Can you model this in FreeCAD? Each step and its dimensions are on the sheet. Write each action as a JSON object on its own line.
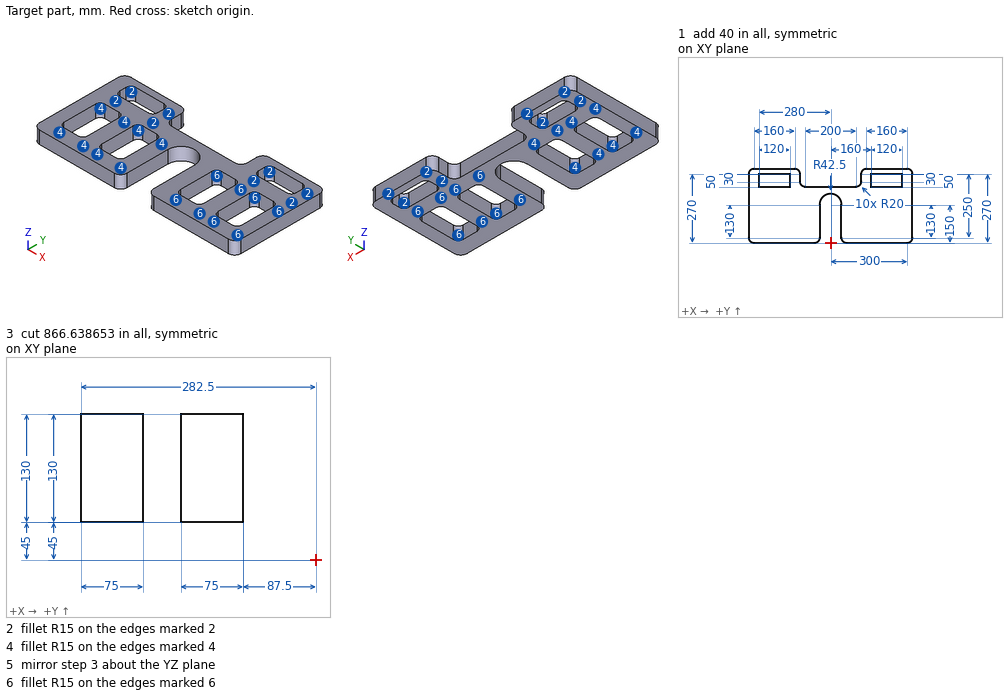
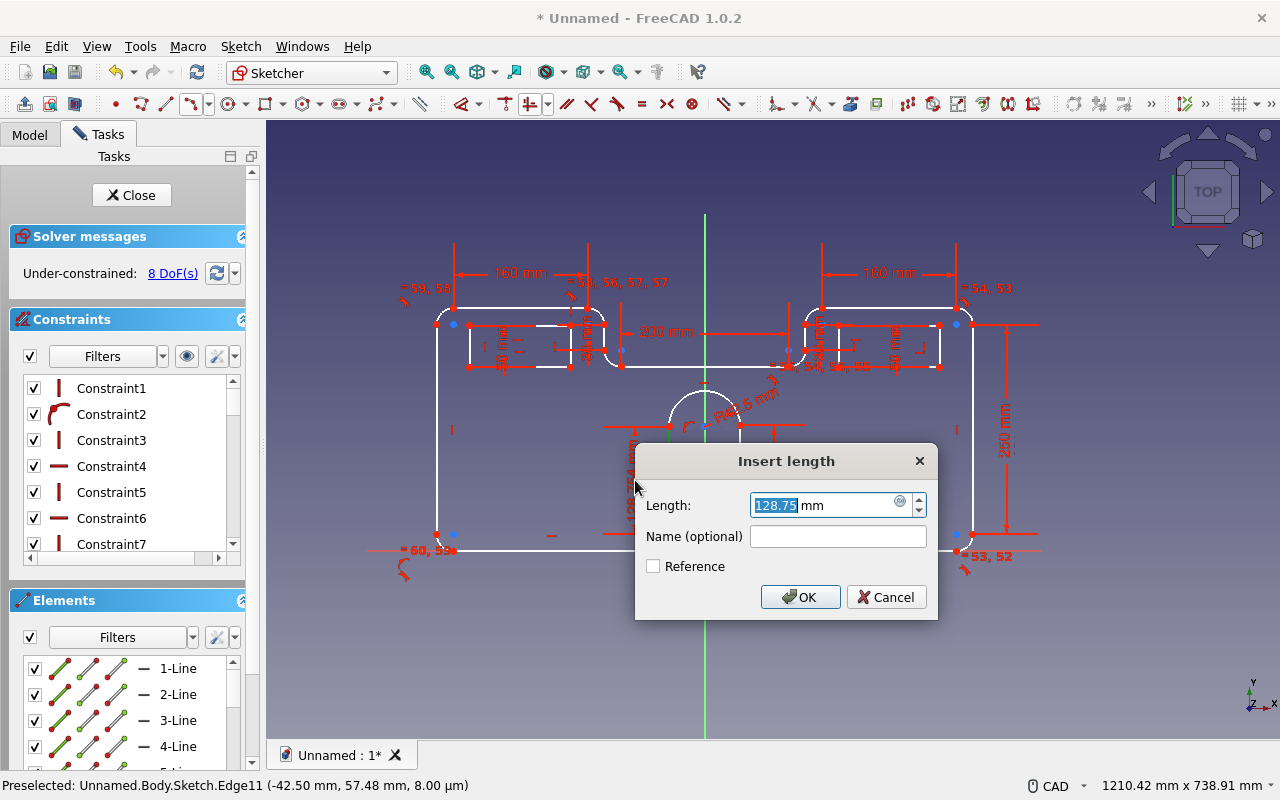
{"action": "type", "text": "130"}
{"action": "key", "text": "Return"}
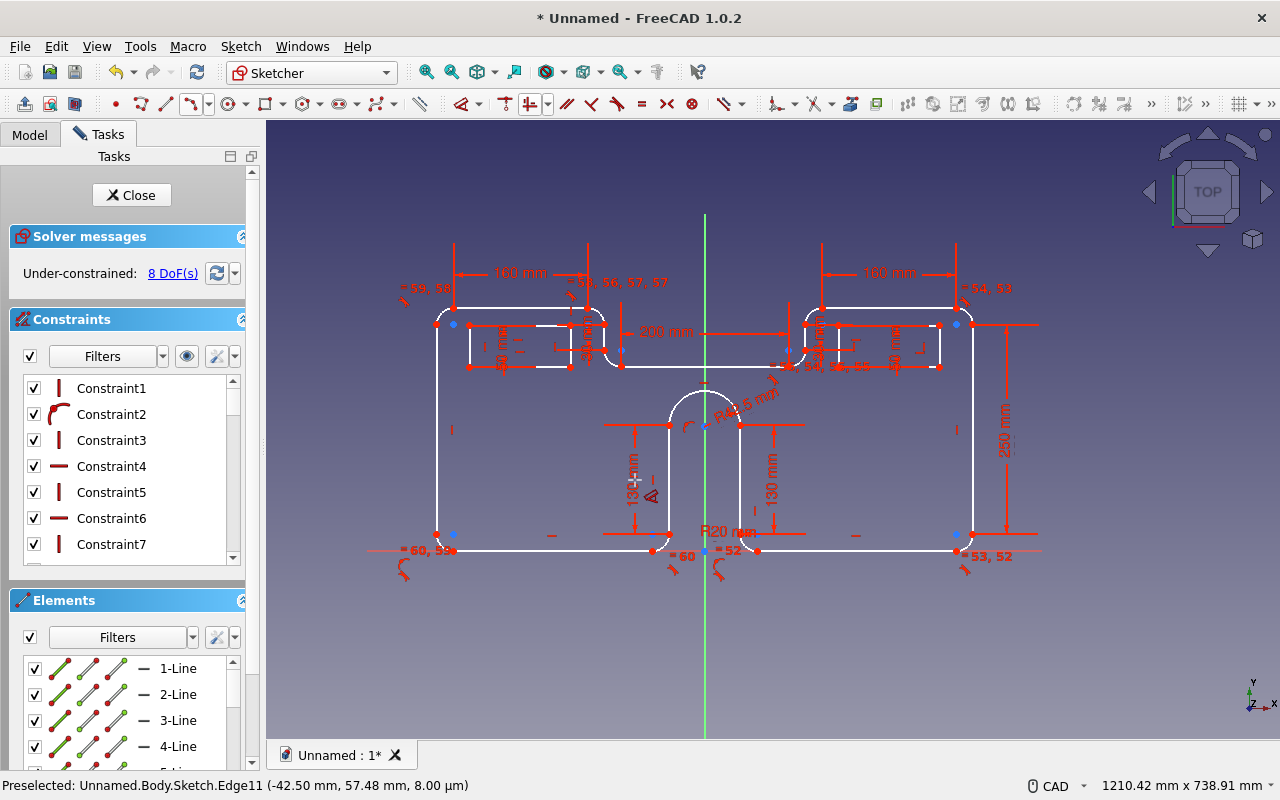
{"action": "left_click", "coordinate": [500, 367]}
{"action": "left_click", "coordinate": [520, 401]}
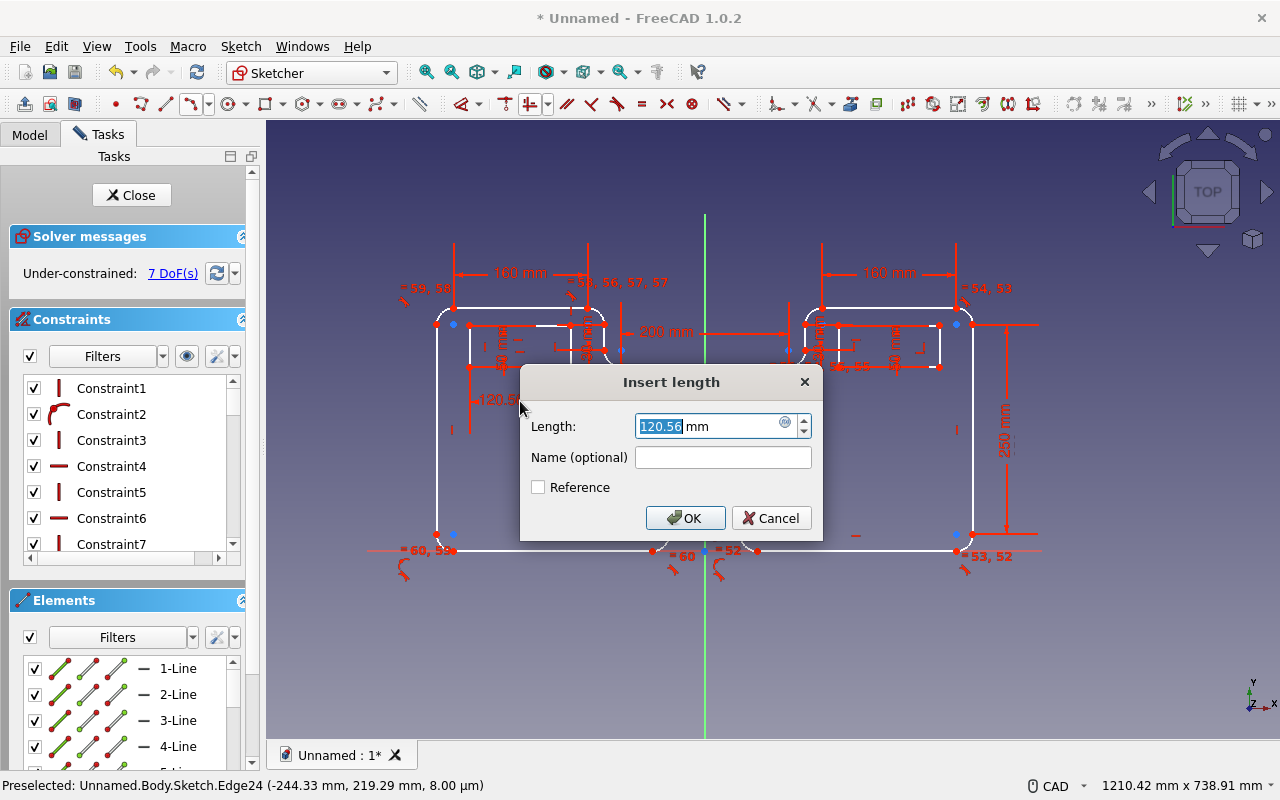
{"action": "type", "text": "120"}
{"action": "key", "text": "Return"}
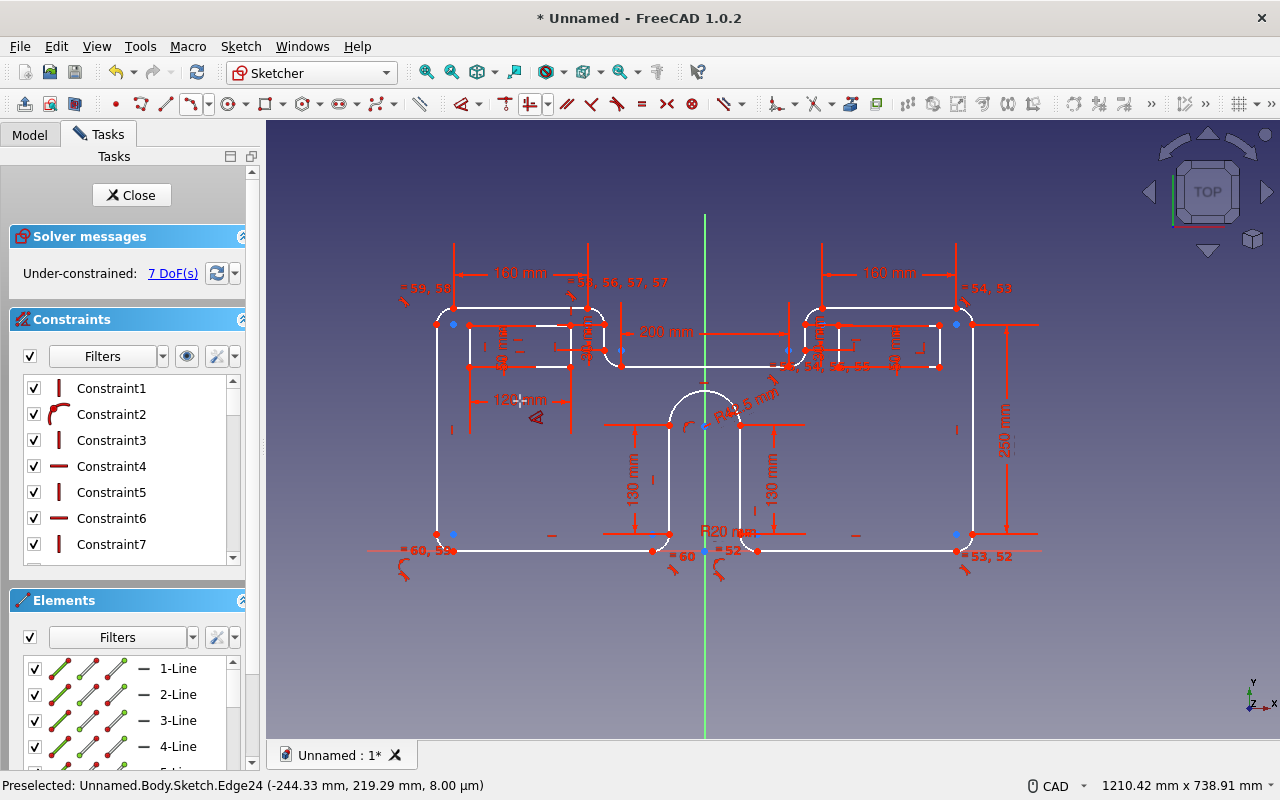
{"action": "left_click", "coordinate": [869, 367]}
{"action": "left_click", "coordinate": [889, 401]}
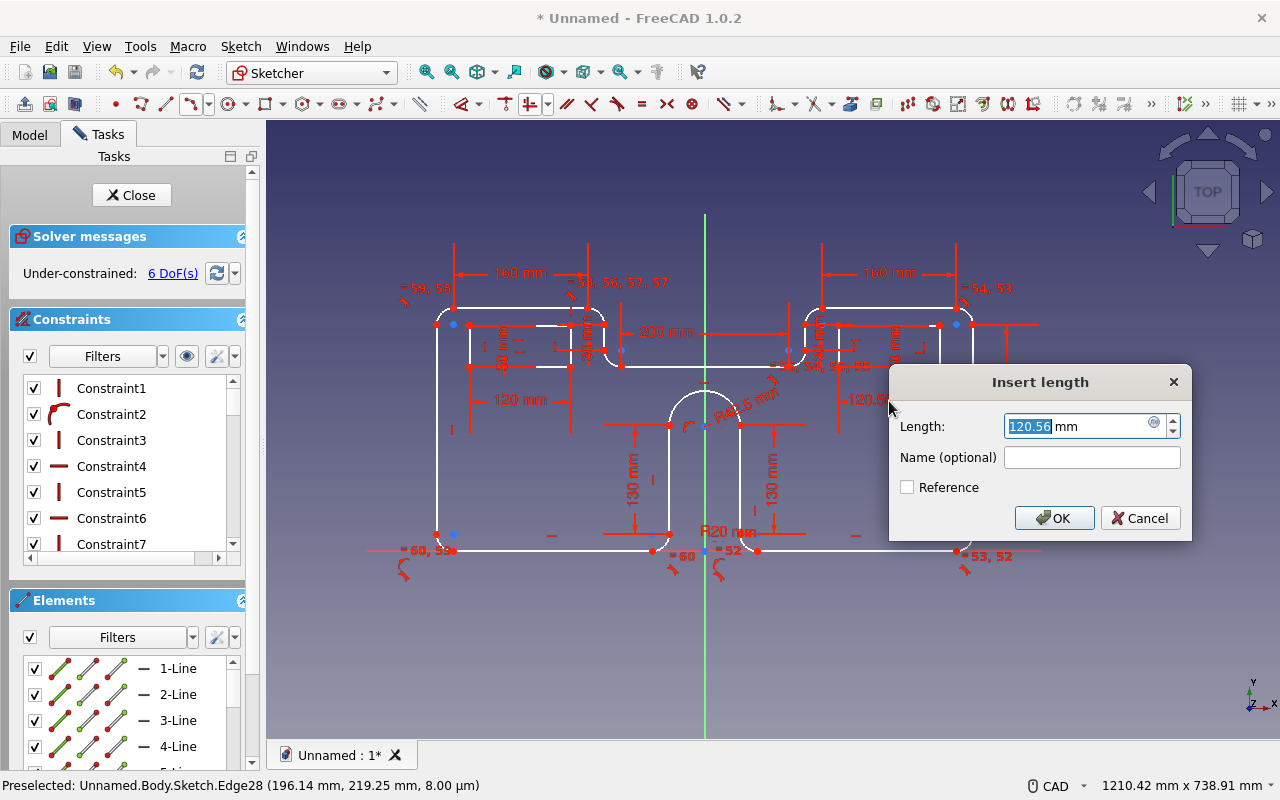
{"action": "type", "text": "120"}
{"action": "key", "text": "Return"}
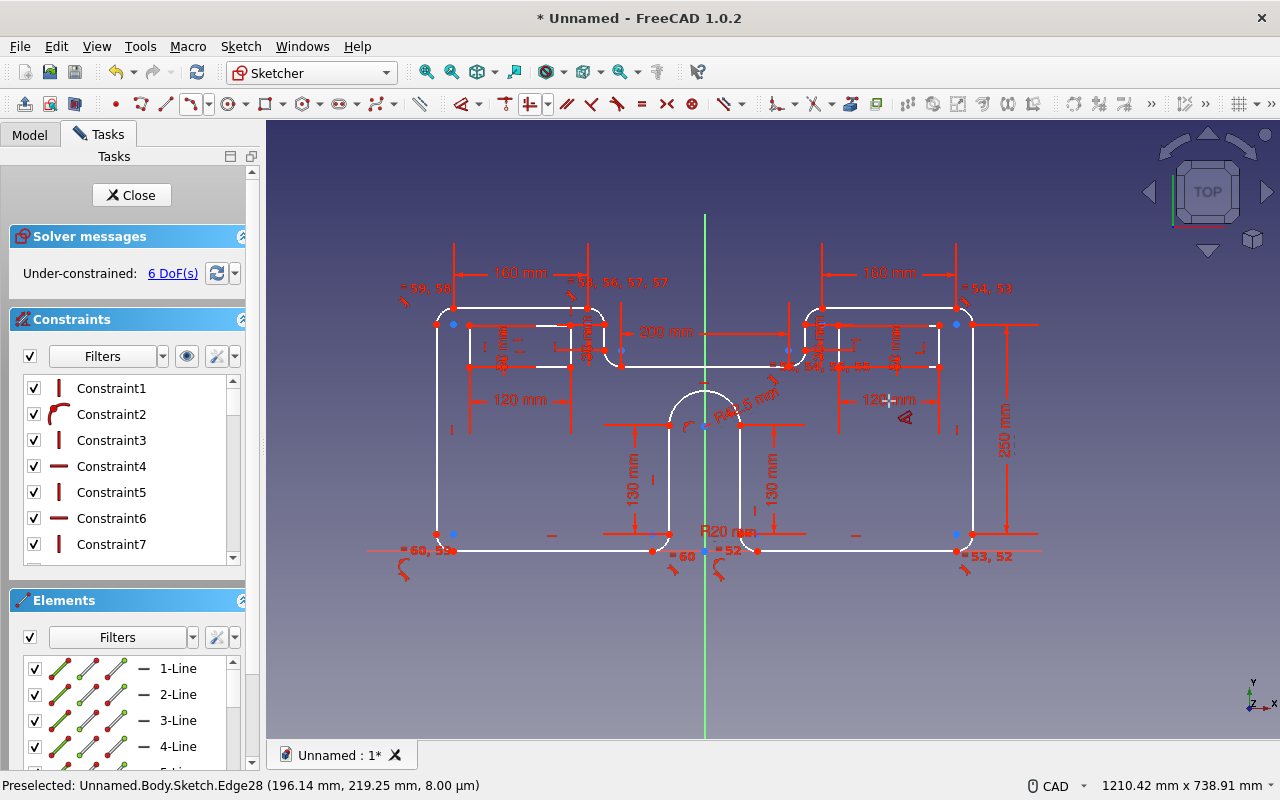
{"action": "left_click", "coordinate": [956, 551]}
{"action": "left_click", "coordinate": [830, 585]}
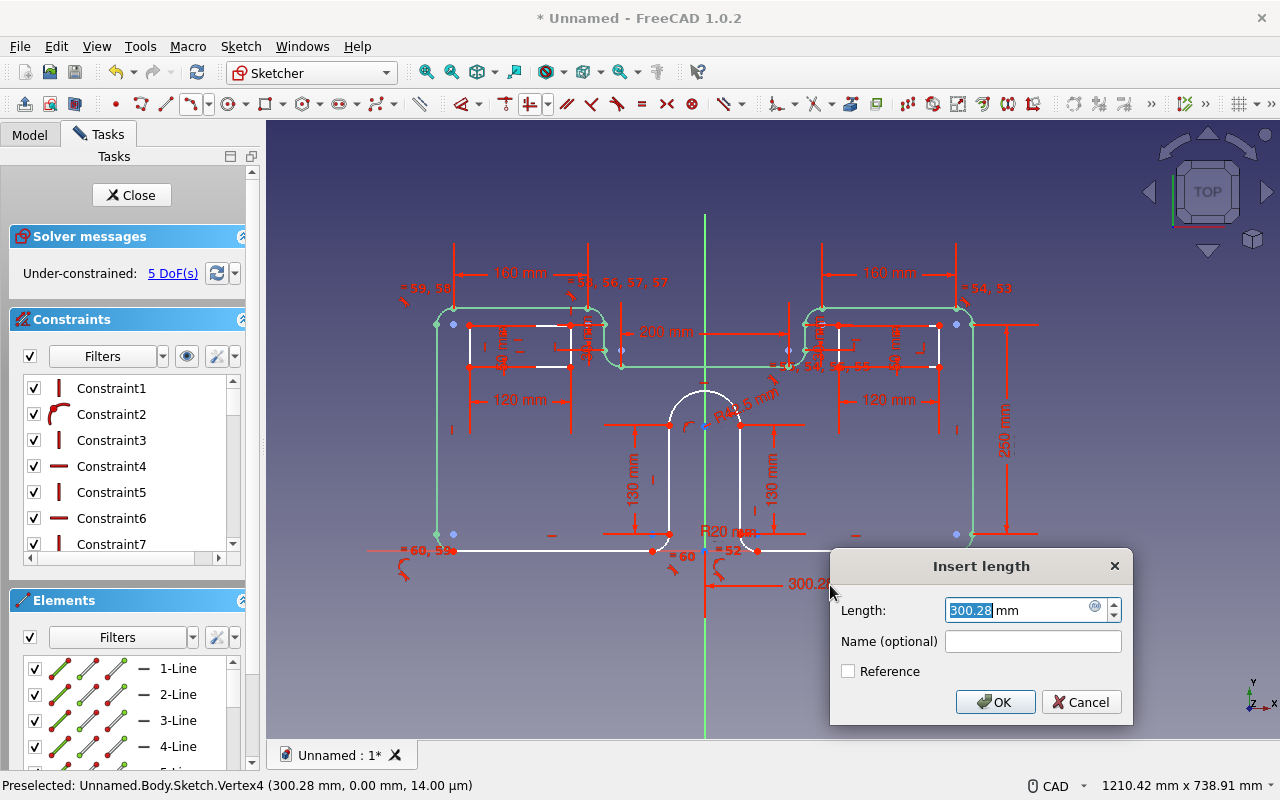
{"action": "type", "text": "300"}
{"action": "key", "text": "Return"}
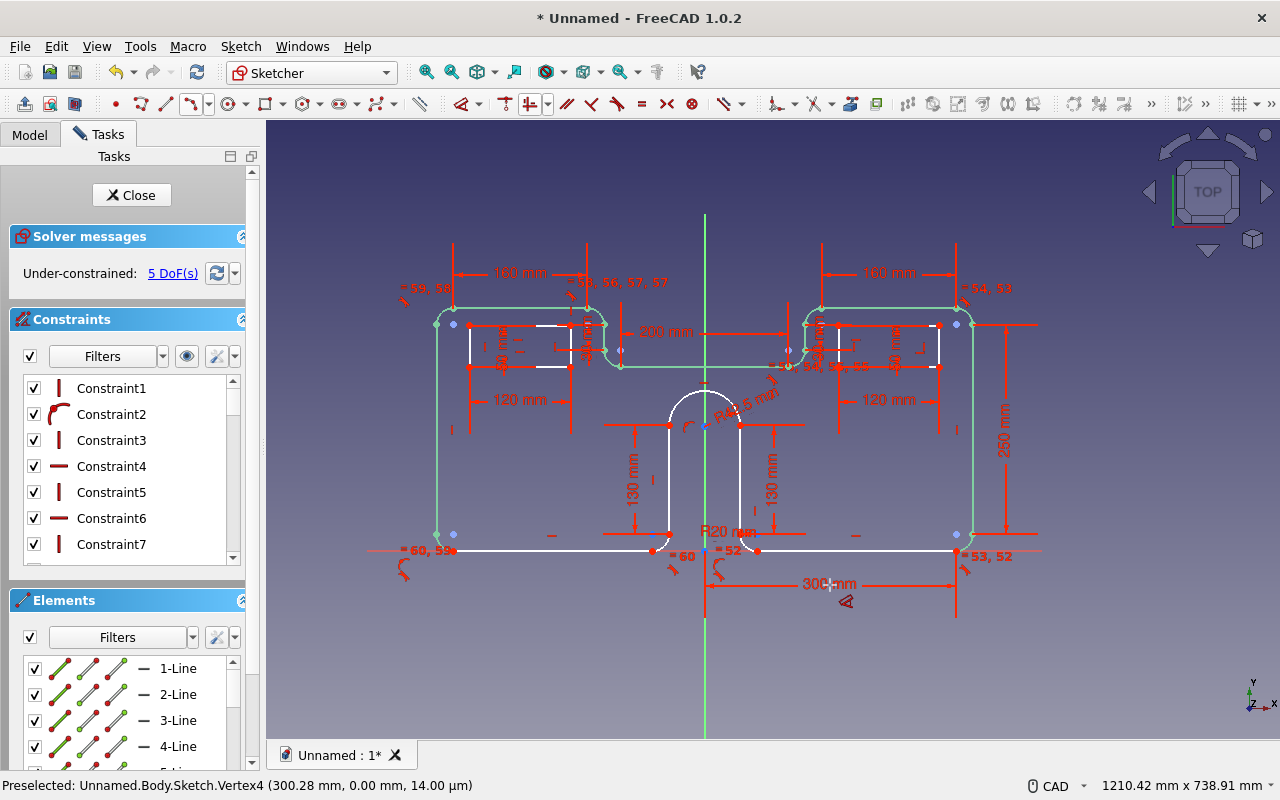
{"action": "left_click", "coordinate": [470, 326]}
{"action": "left_click", "coordinate": [587, 585]}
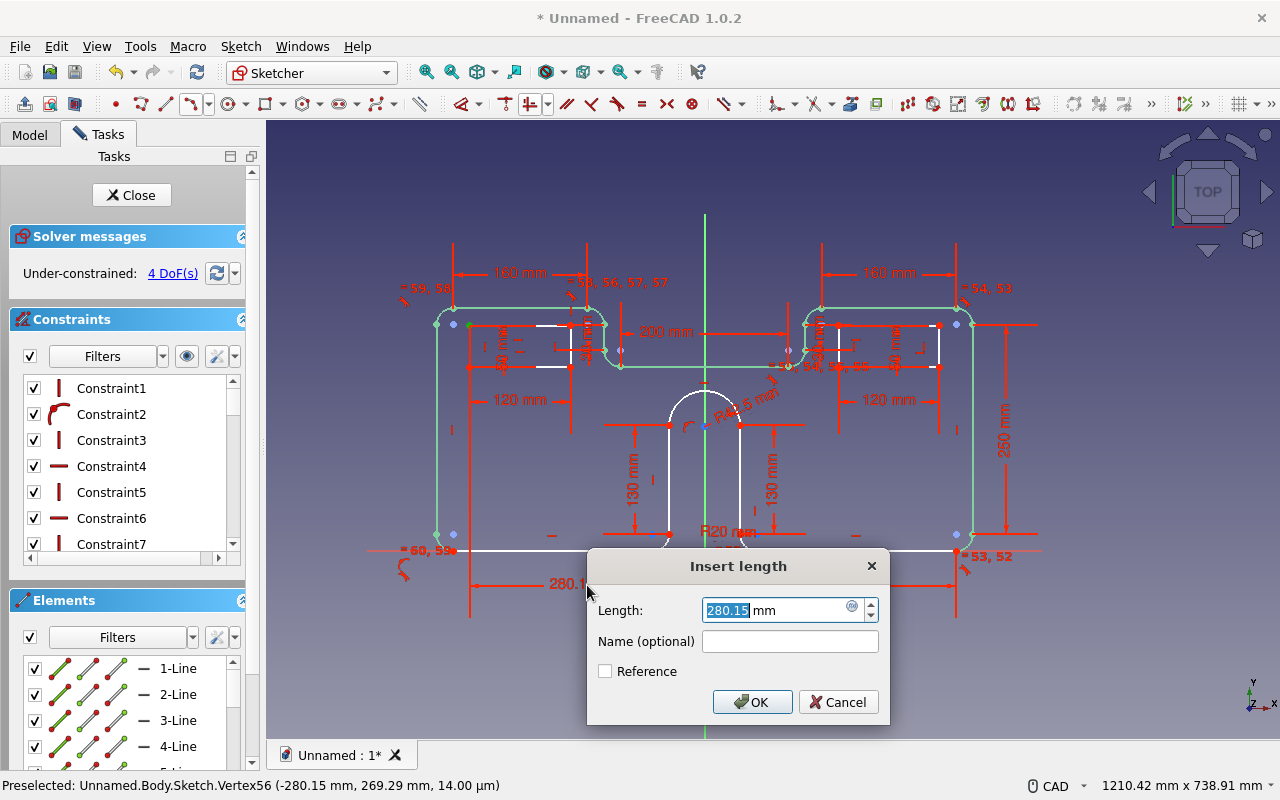
{"action": "type", "text": "280"}
{"action": "key", "text": "Return"}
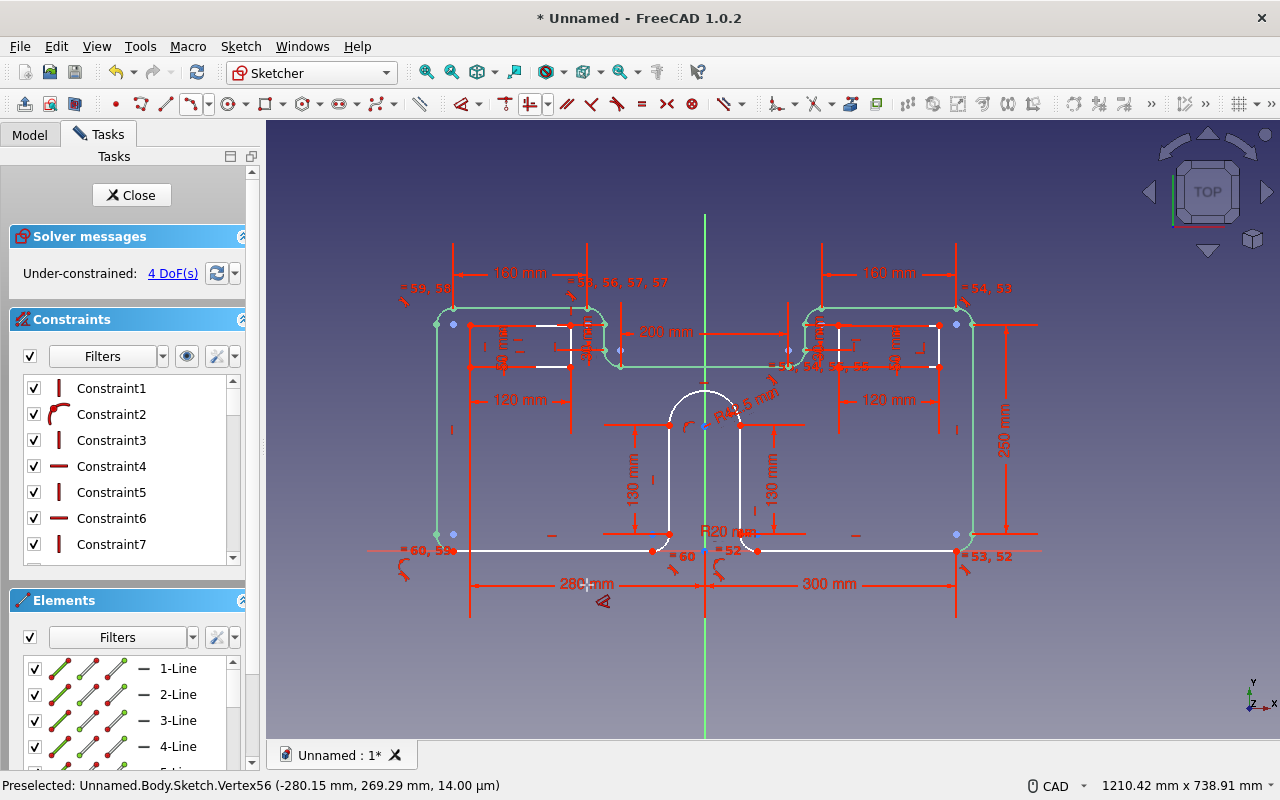
{"action": "left_click", "coordinate": [470, 326]}
{"action": "left_click", "coordinate": [412, 438]}